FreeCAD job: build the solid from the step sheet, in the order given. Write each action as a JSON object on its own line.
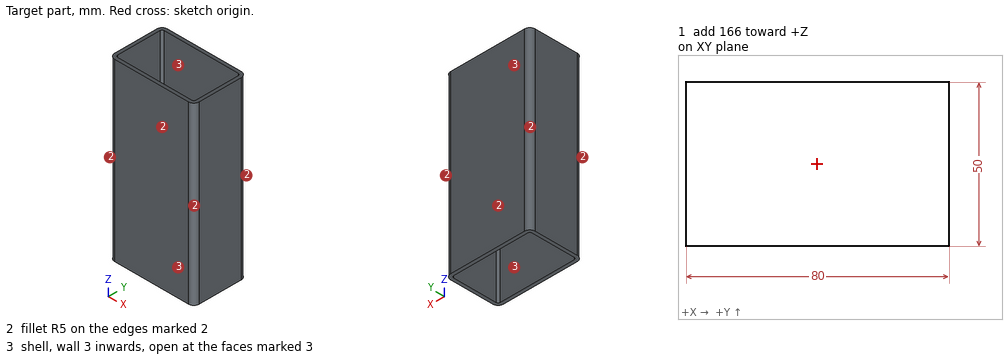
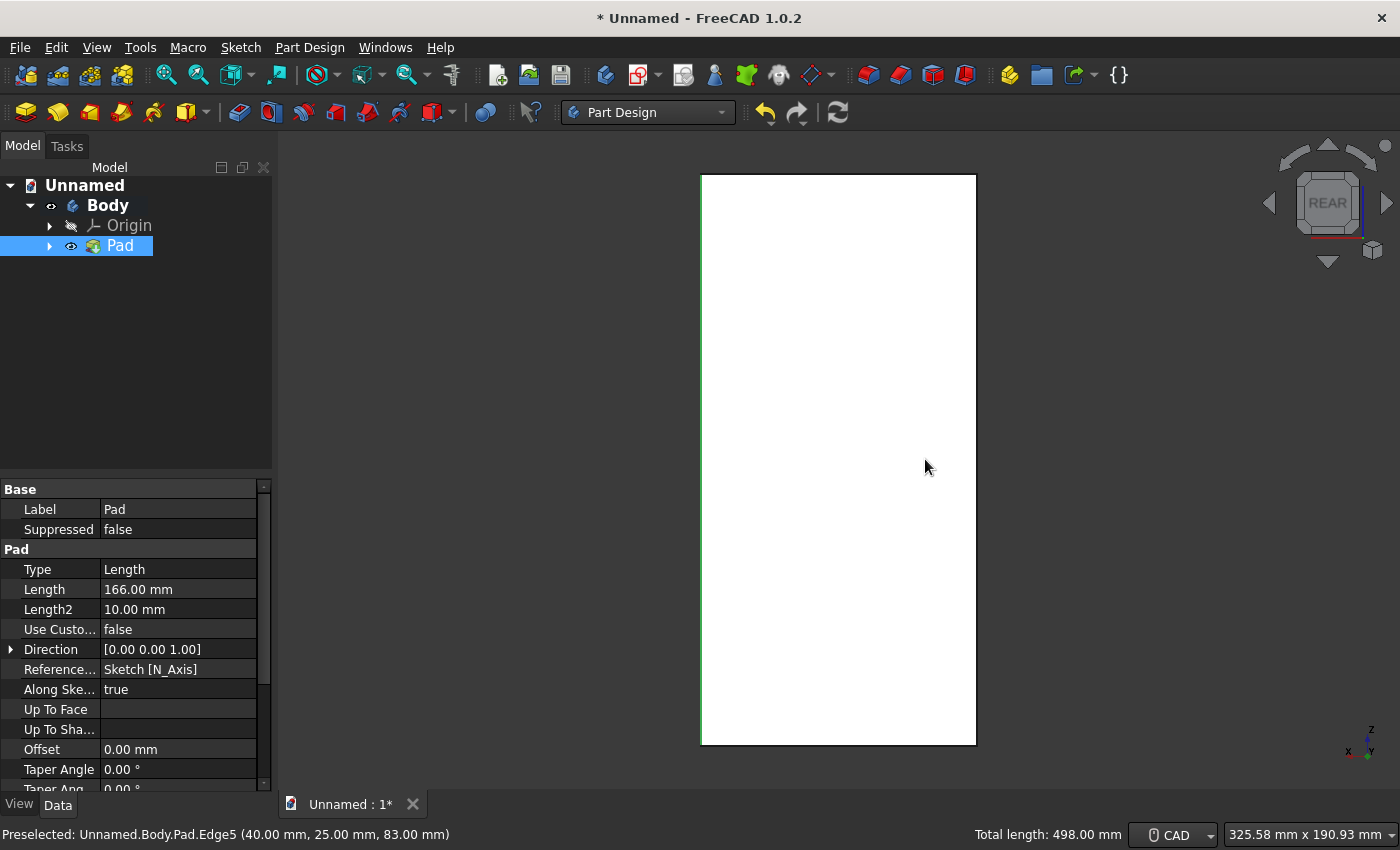
{"action": "left_click", "coordinate": [977, 459], "text": "ctrl"}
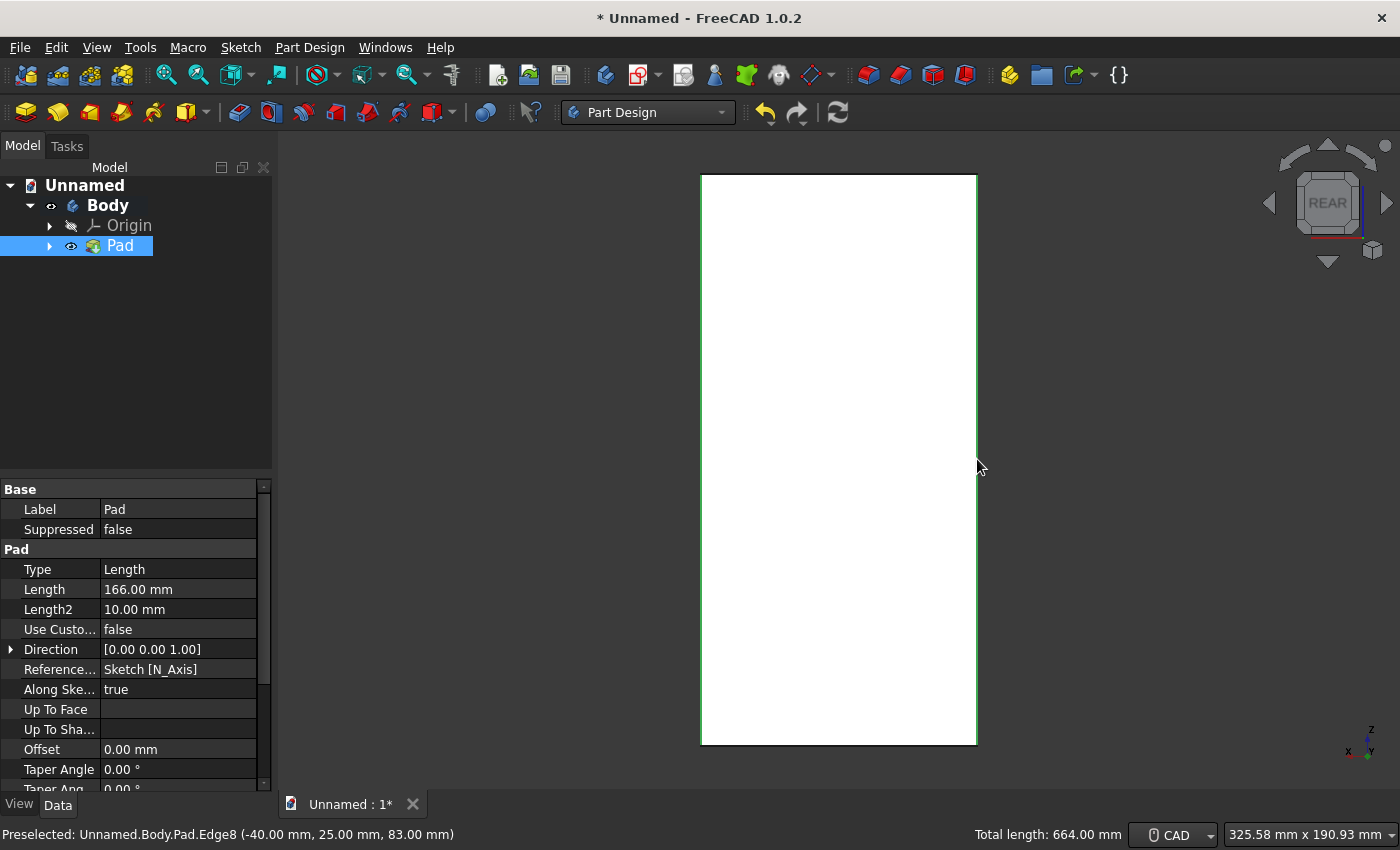
{"action": "left_click", "coordinate": [870, 76]}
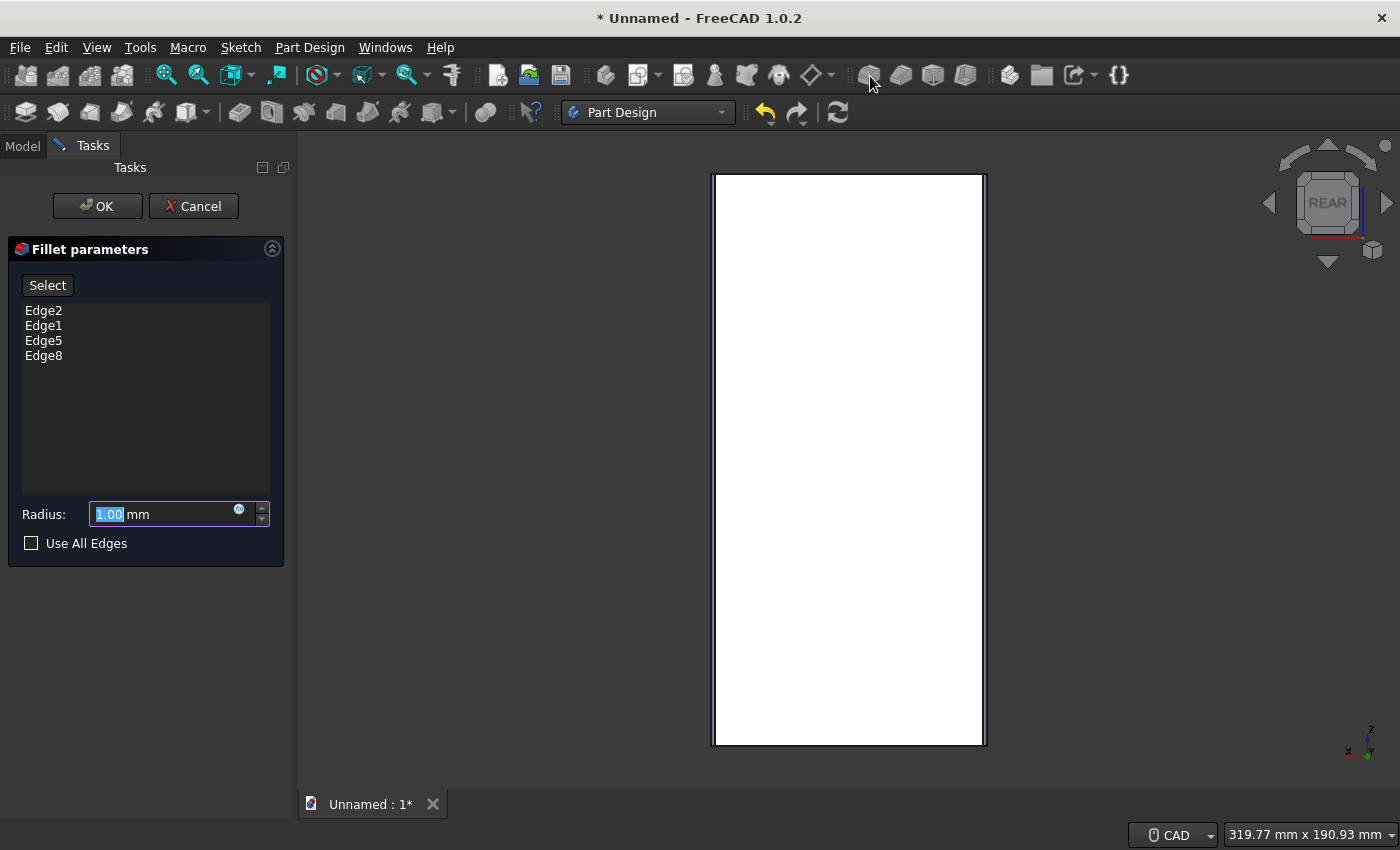
{"action": "type", "text": "5"}
{"action": "key", "text": "Tab"}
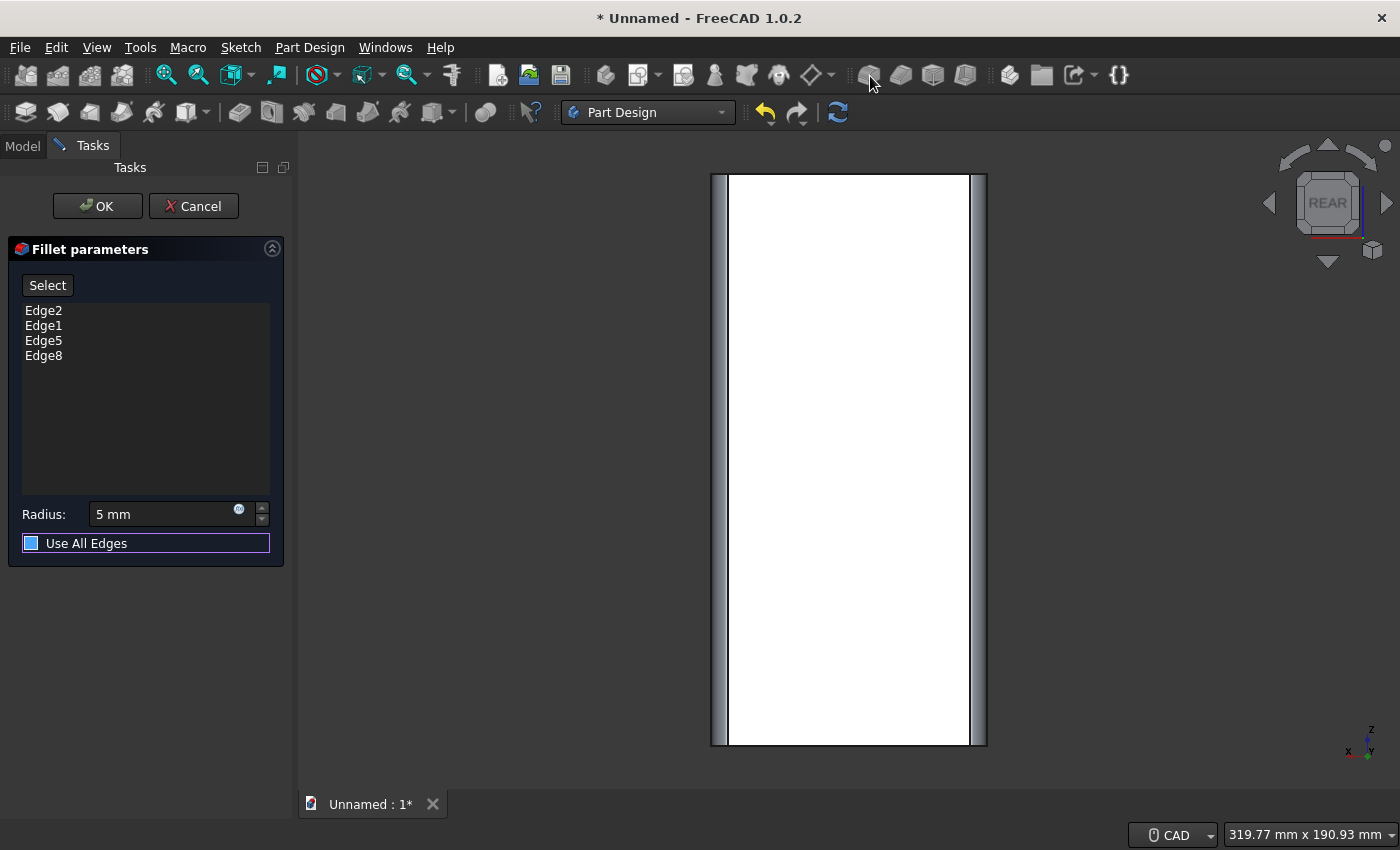
{"action": "left_click", "coordinate": [98, 206]}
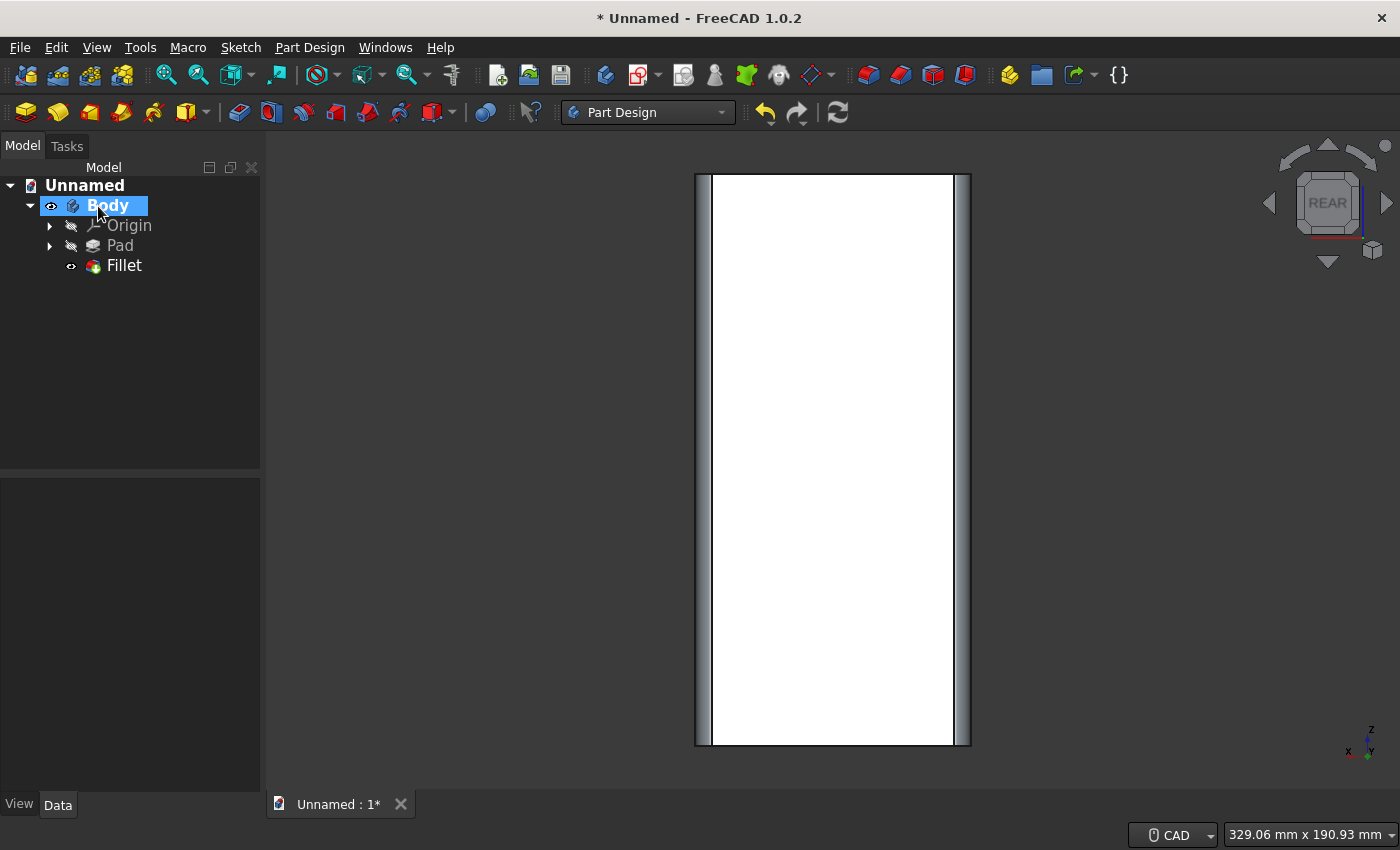
{"action": "key", "text": "0"}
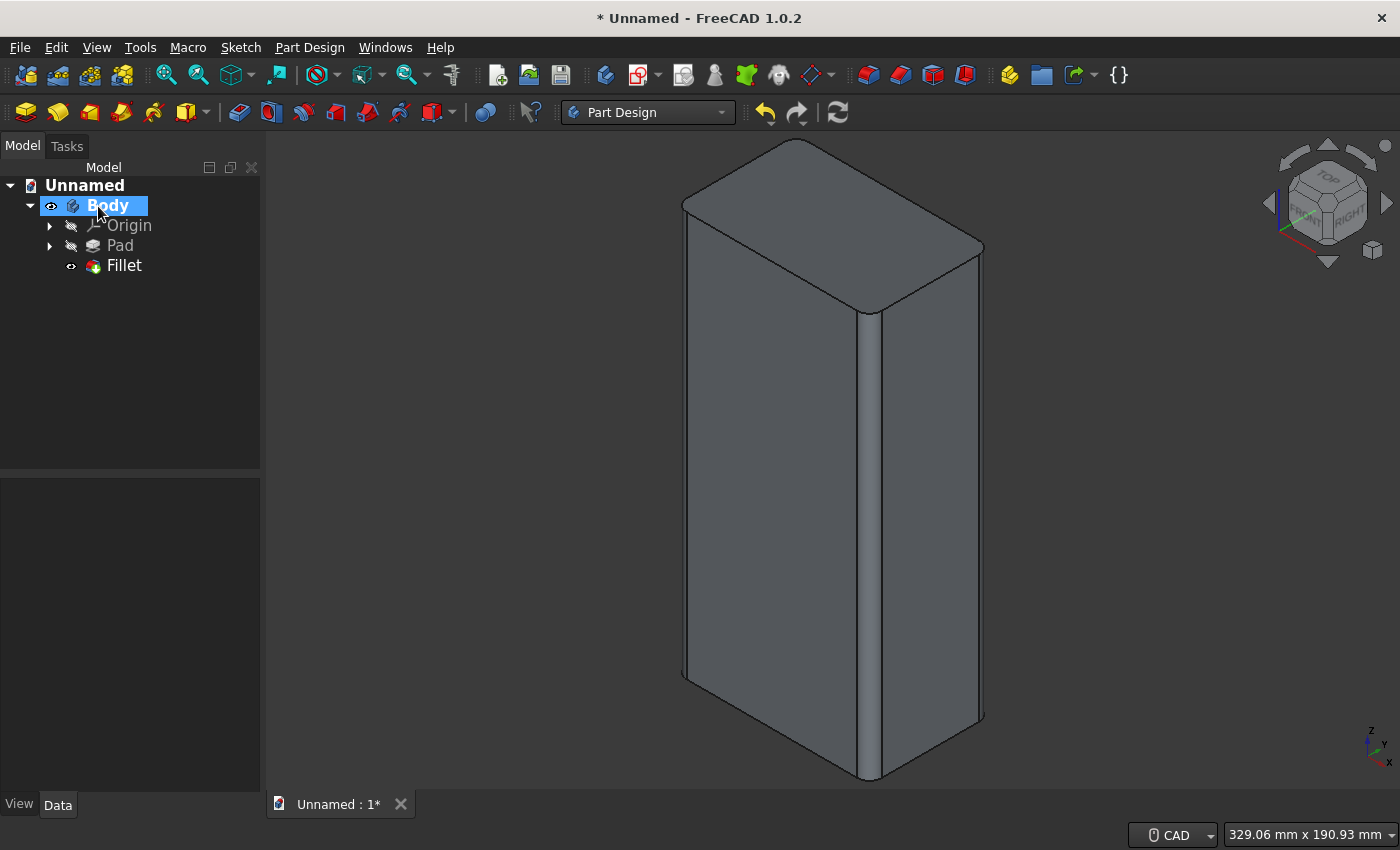
{"action": "left_click", "coordinate": [861, 242]}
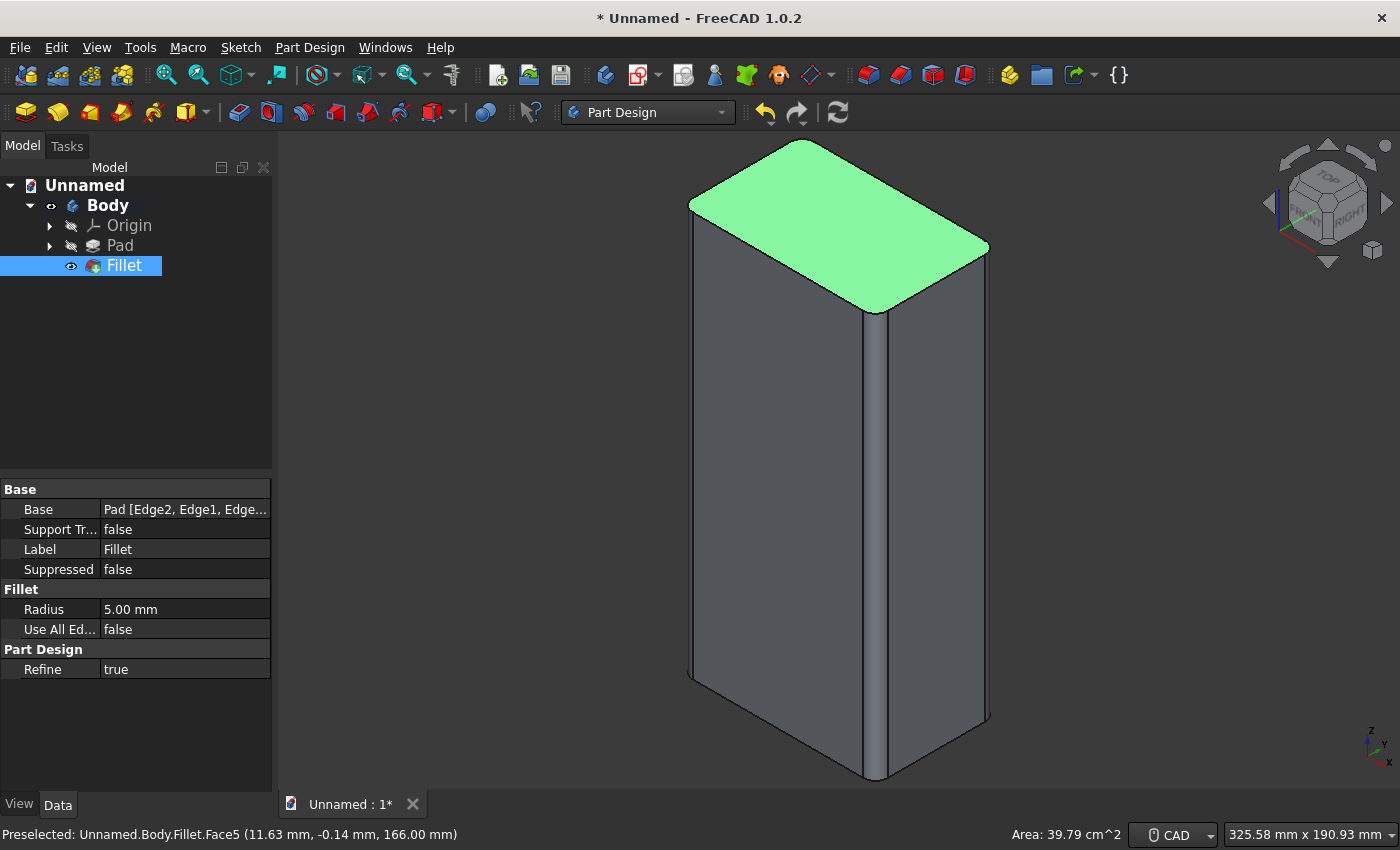
{"action": "key", "text": "2"}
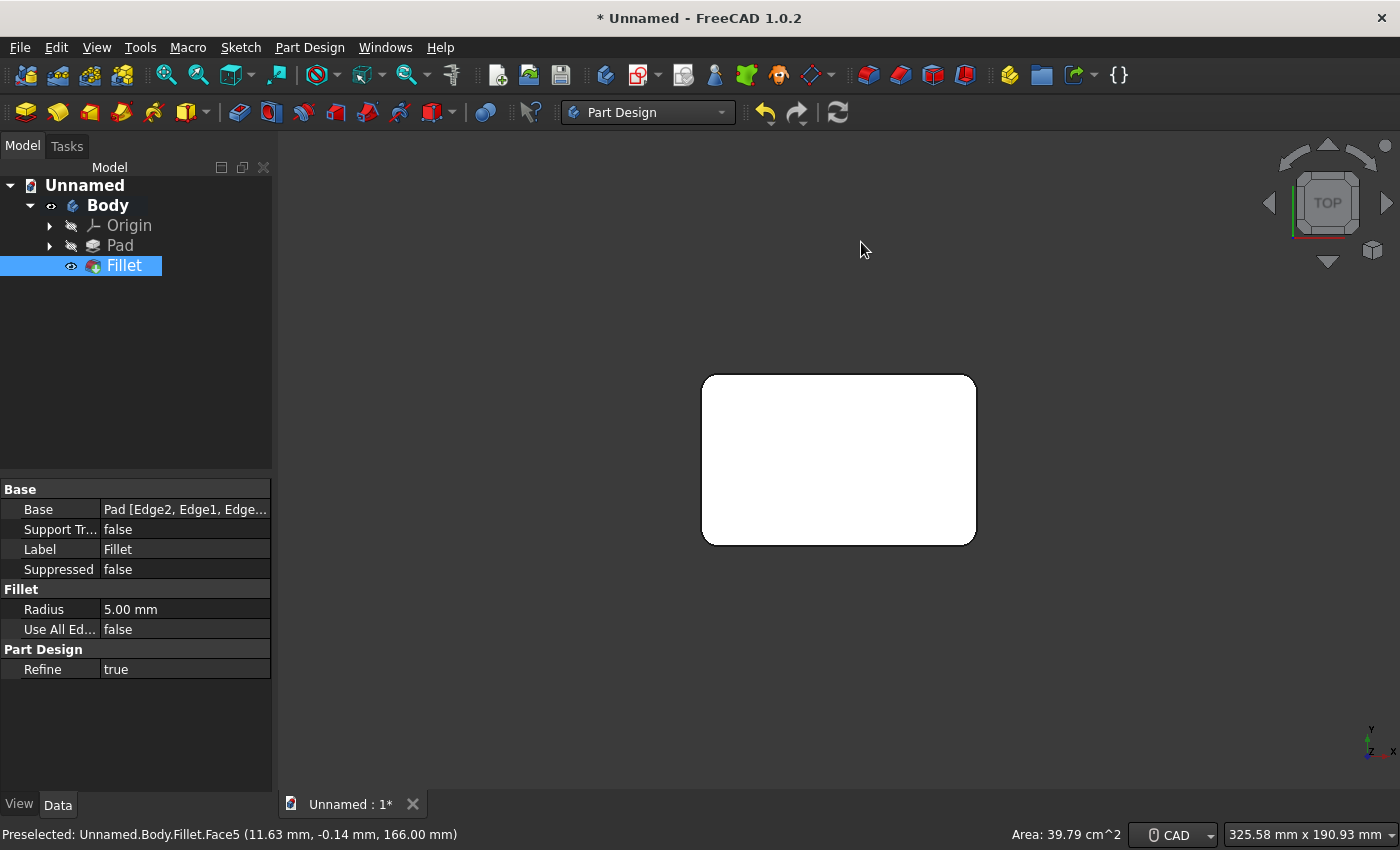
{"action": "key", "text": "v f"}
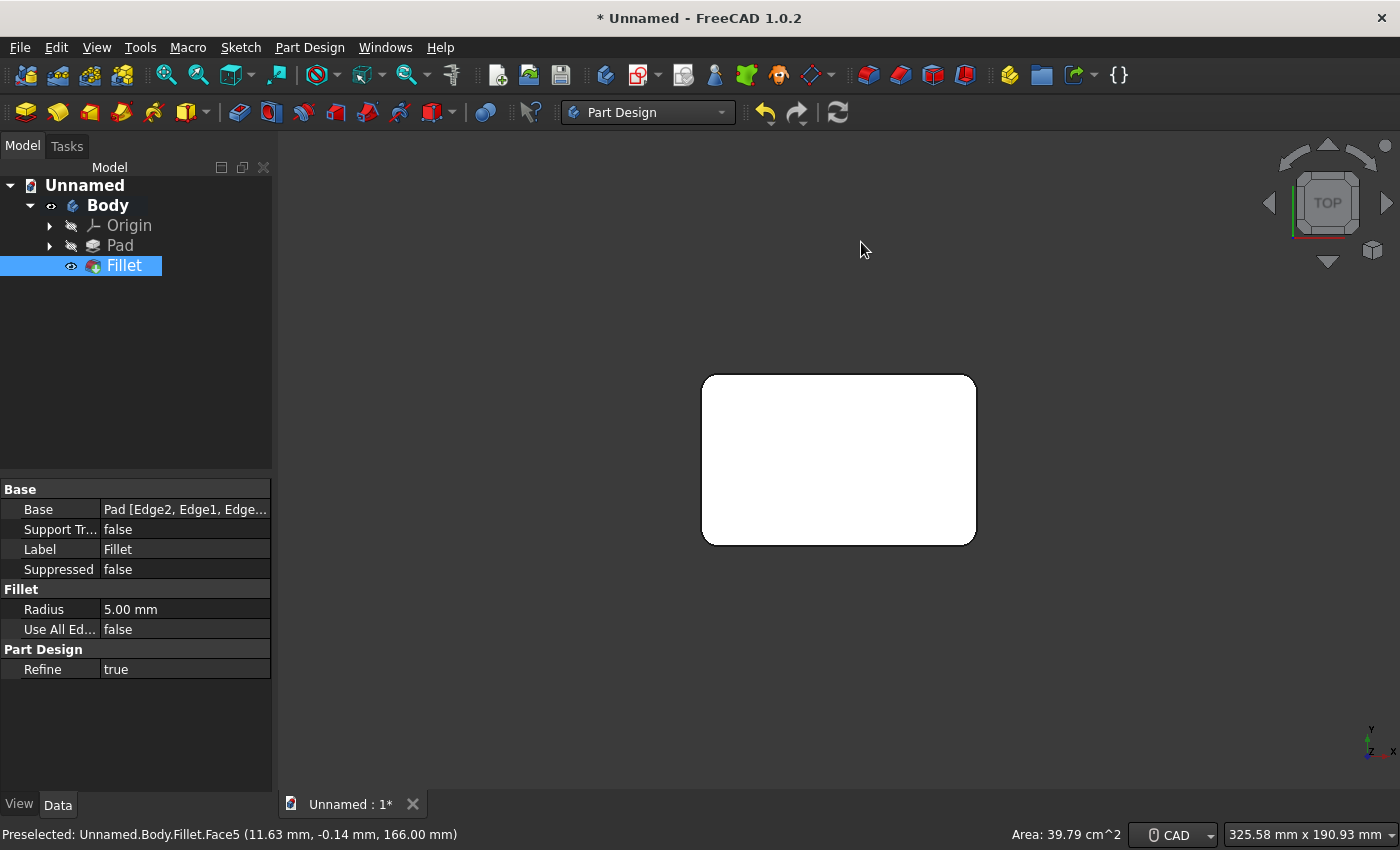
{"action": "key", "text": "1"}